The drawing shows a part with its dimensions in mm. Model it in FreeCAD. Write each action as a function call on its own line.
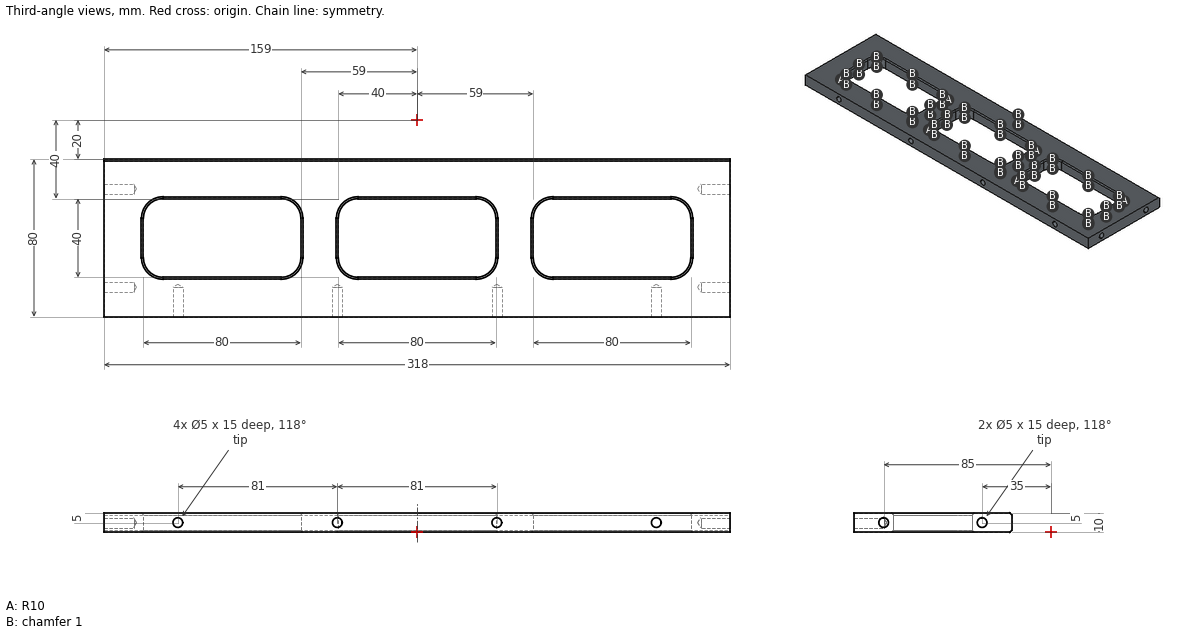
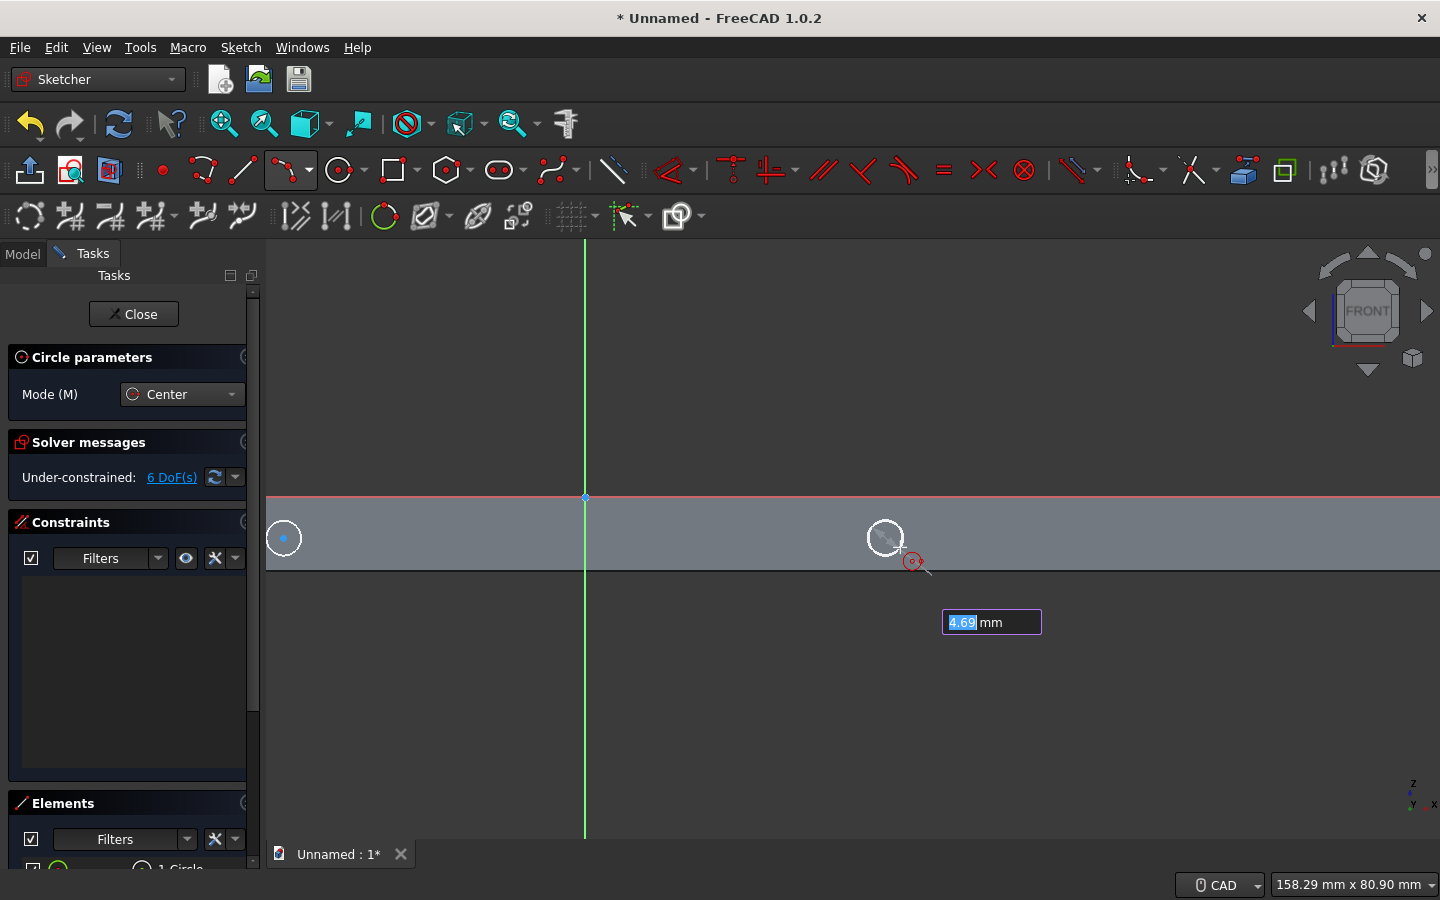
click(898, 547)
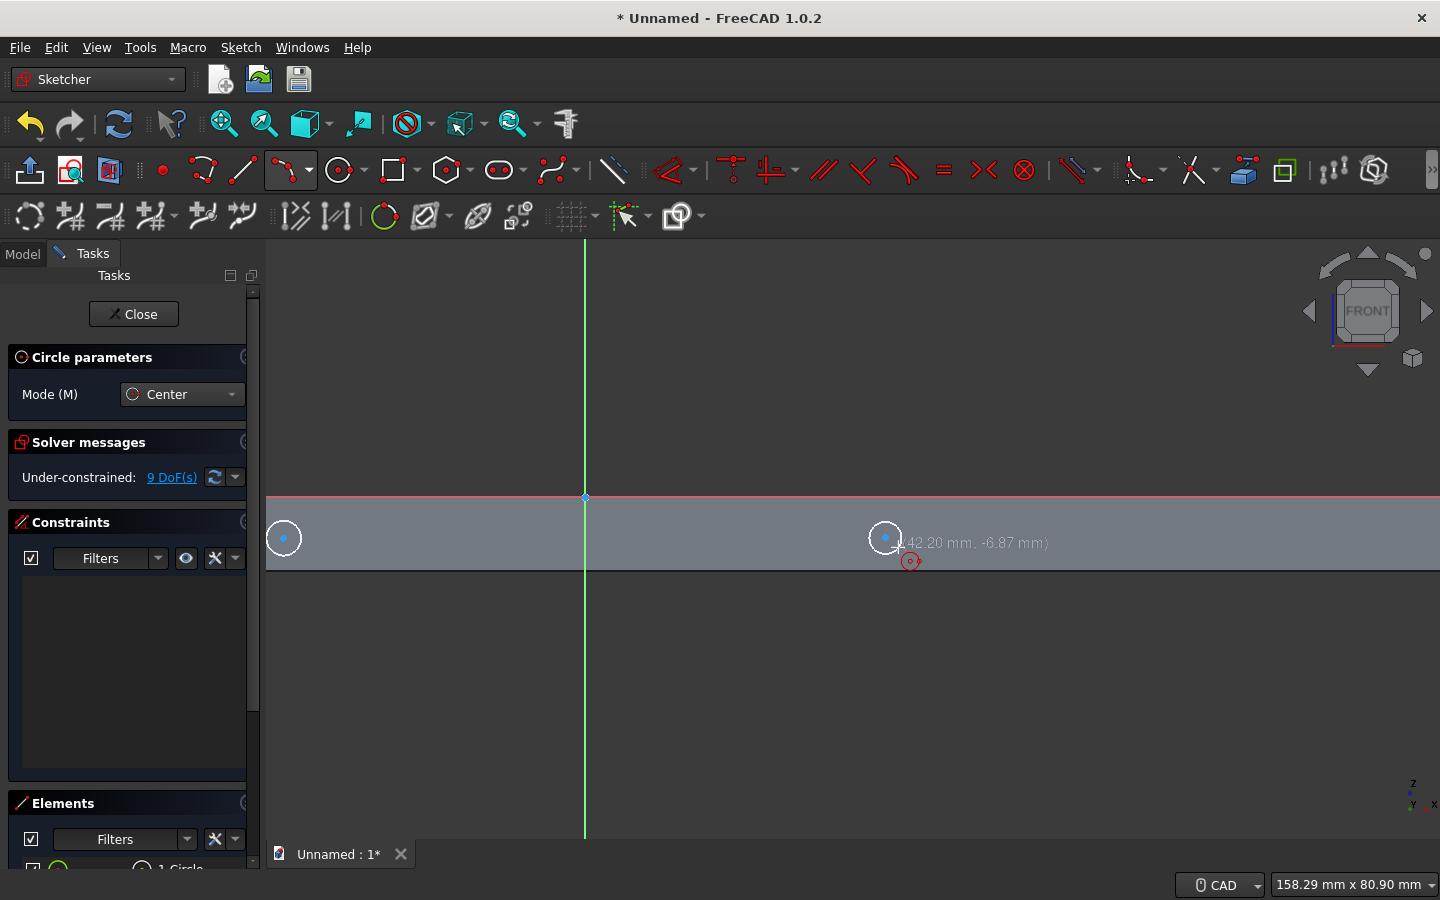
scroll(901, 547, down, 5)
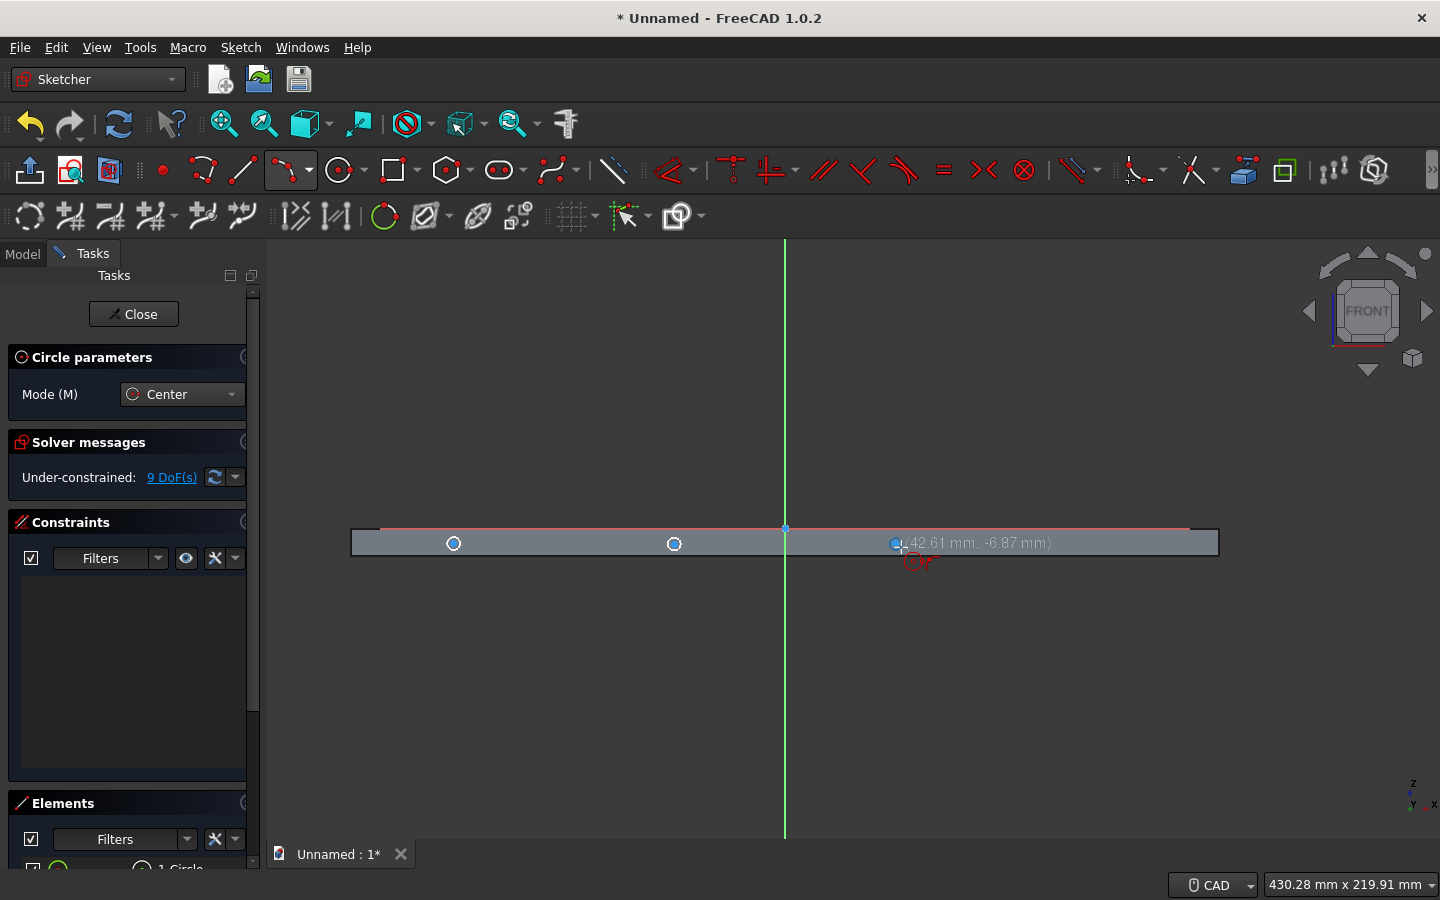
scroll(1117, 543, up, 7)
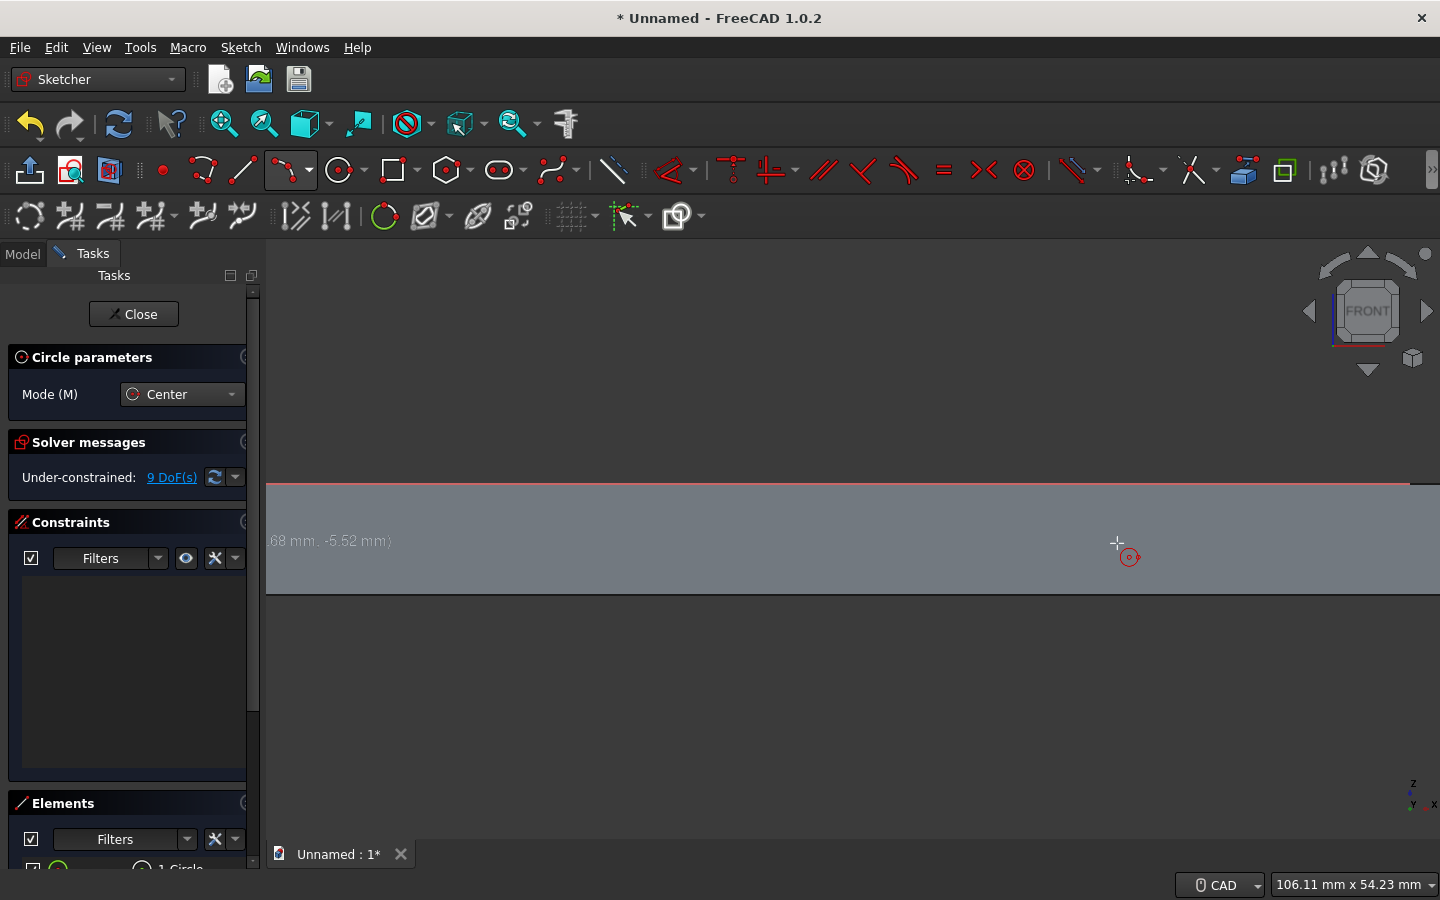
scroll(1117, 543, down, 7)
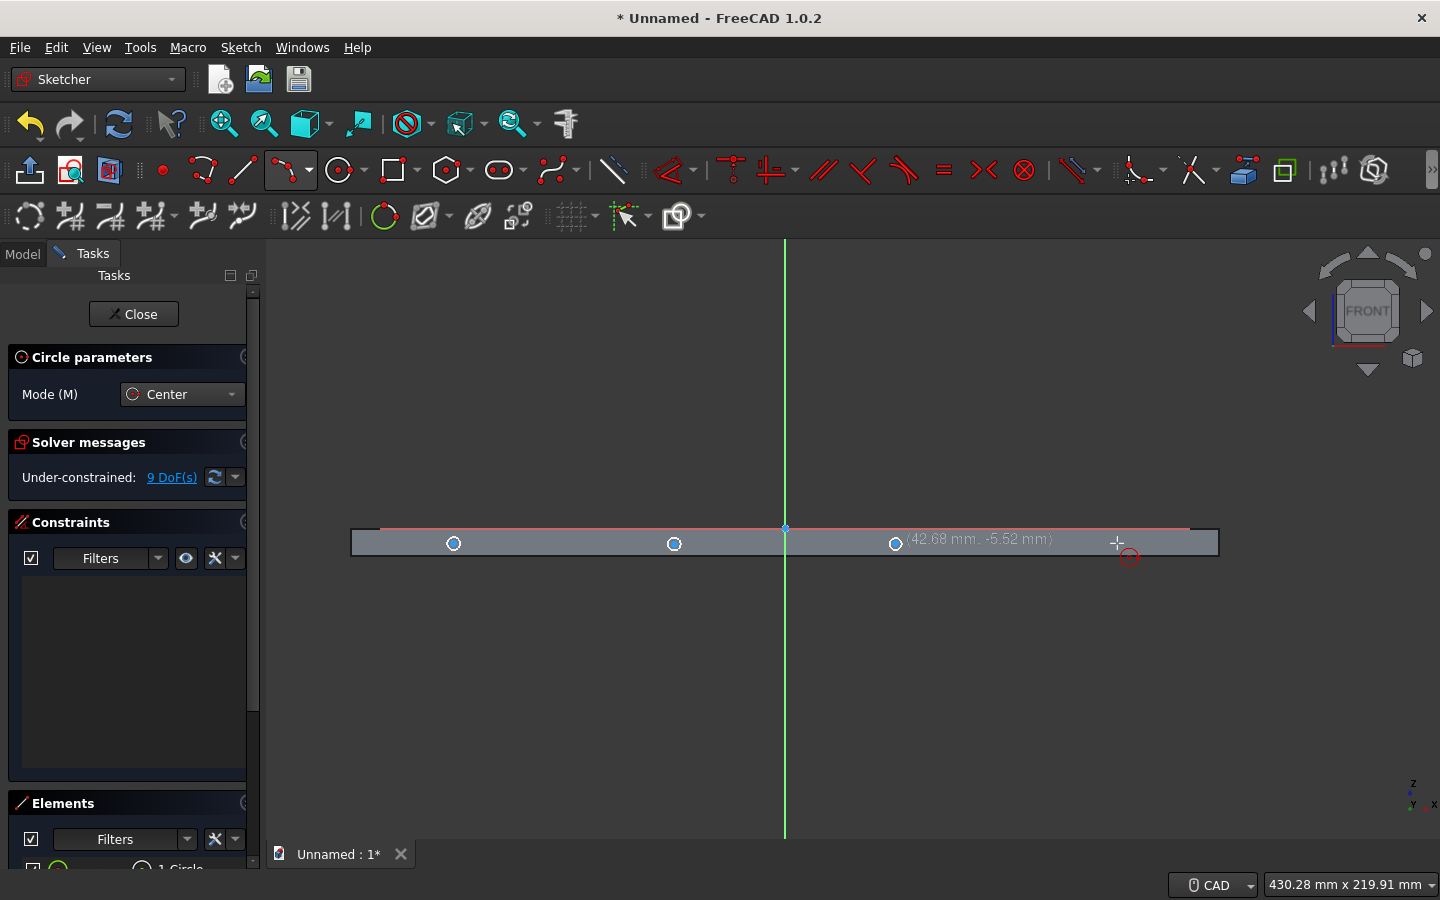
click(1117, 543)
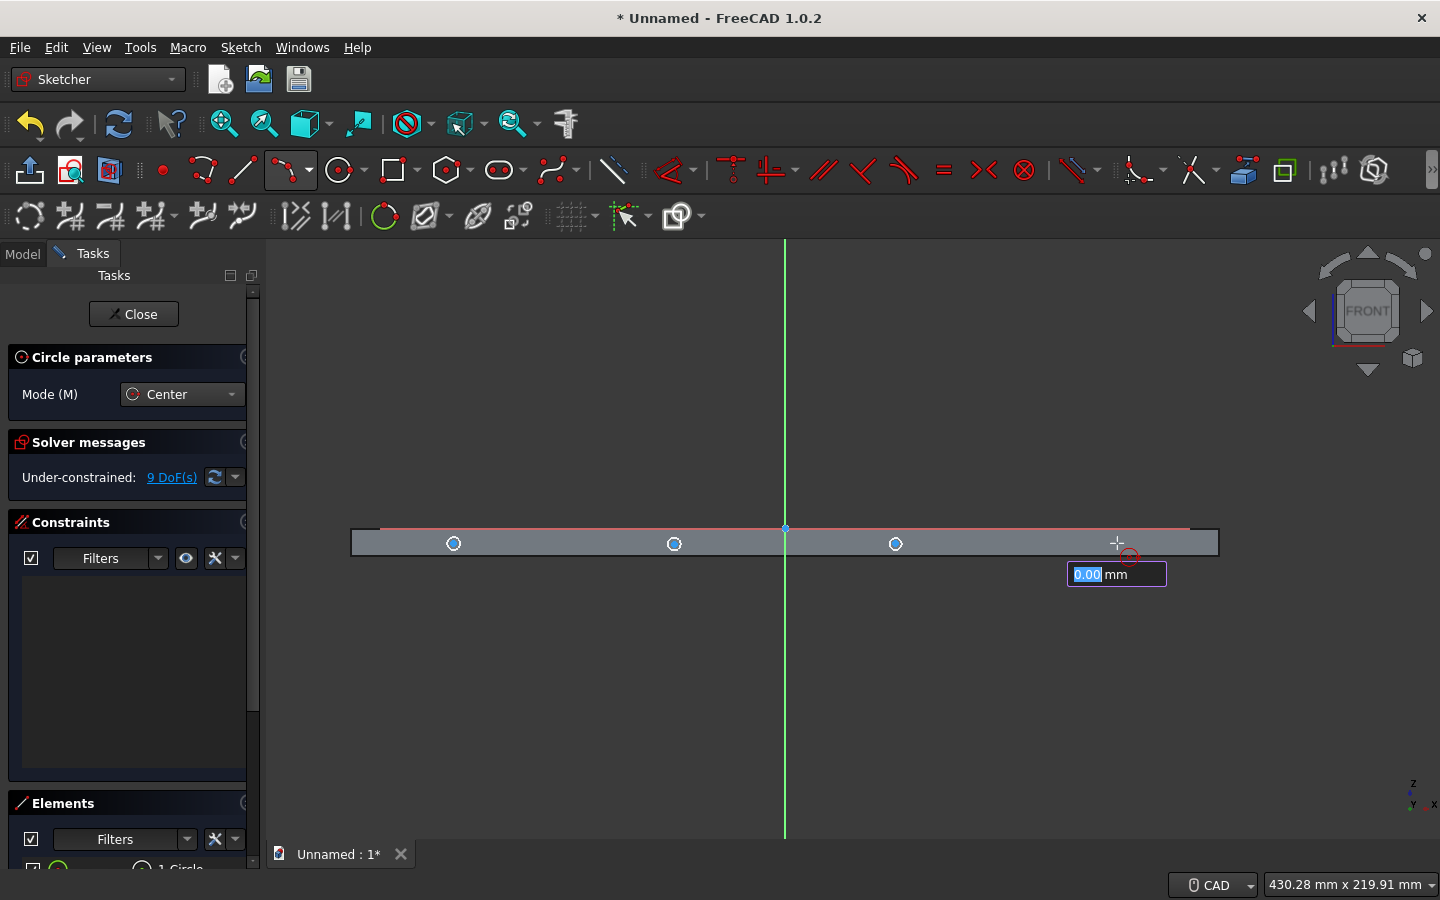
scroll(1121, 547, up, 5)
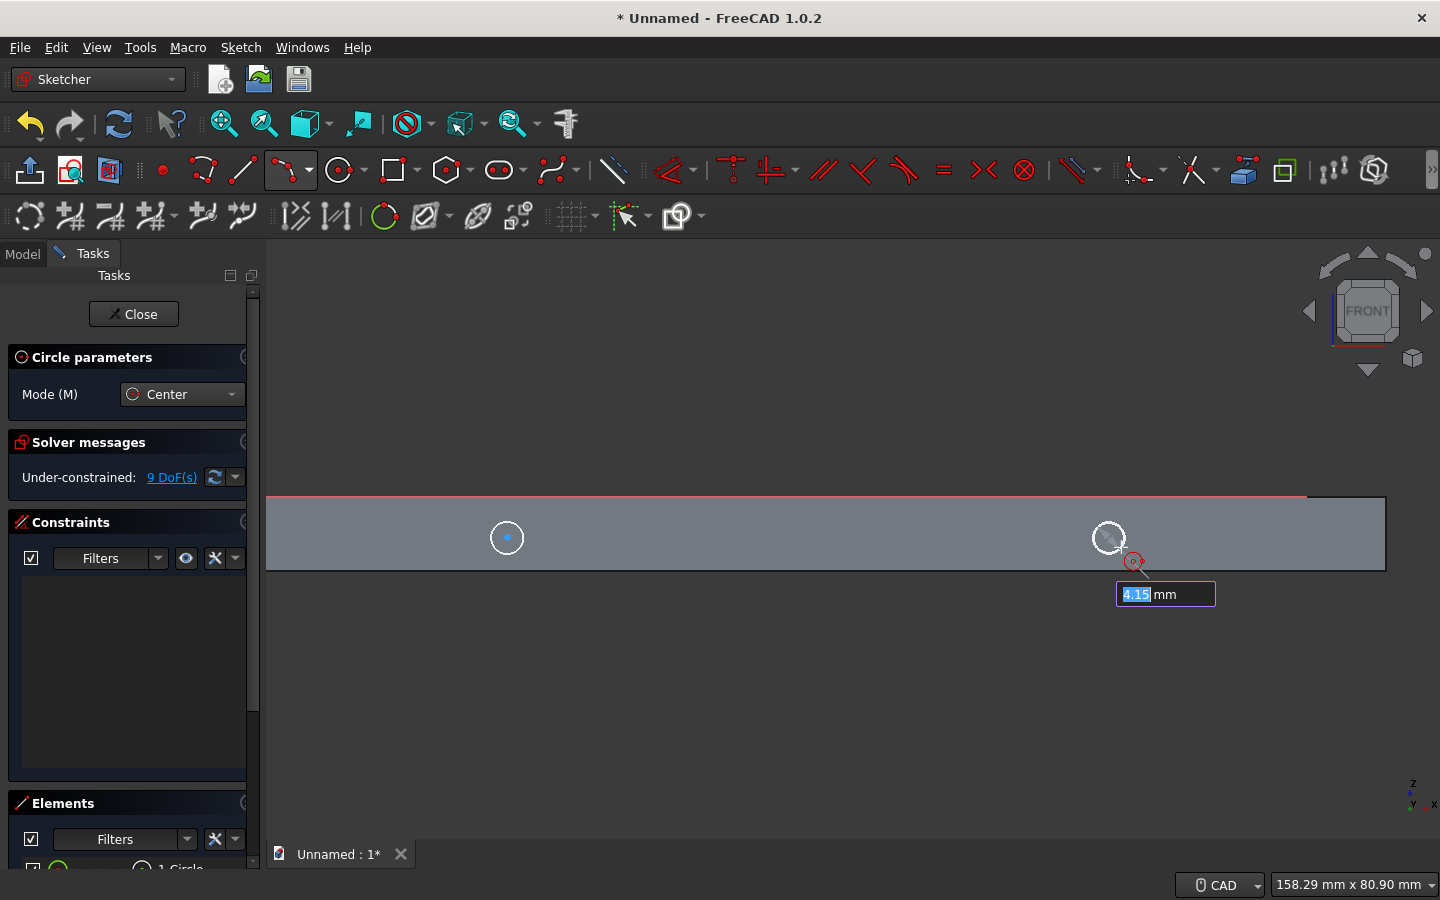
click(1121, 547)
key(Escape)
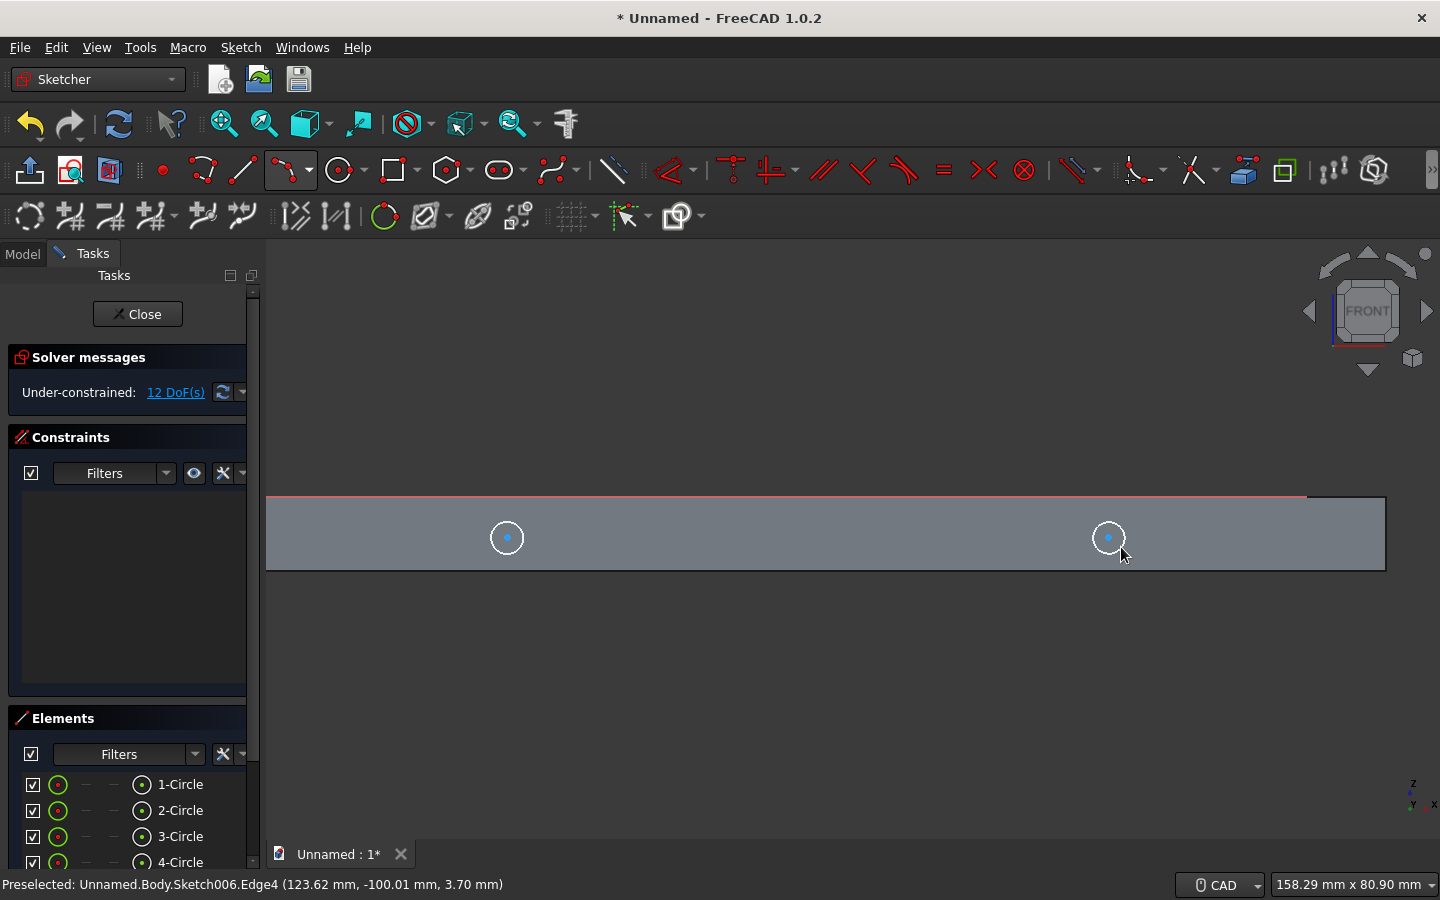
scroll(1121, 547, down, 5)